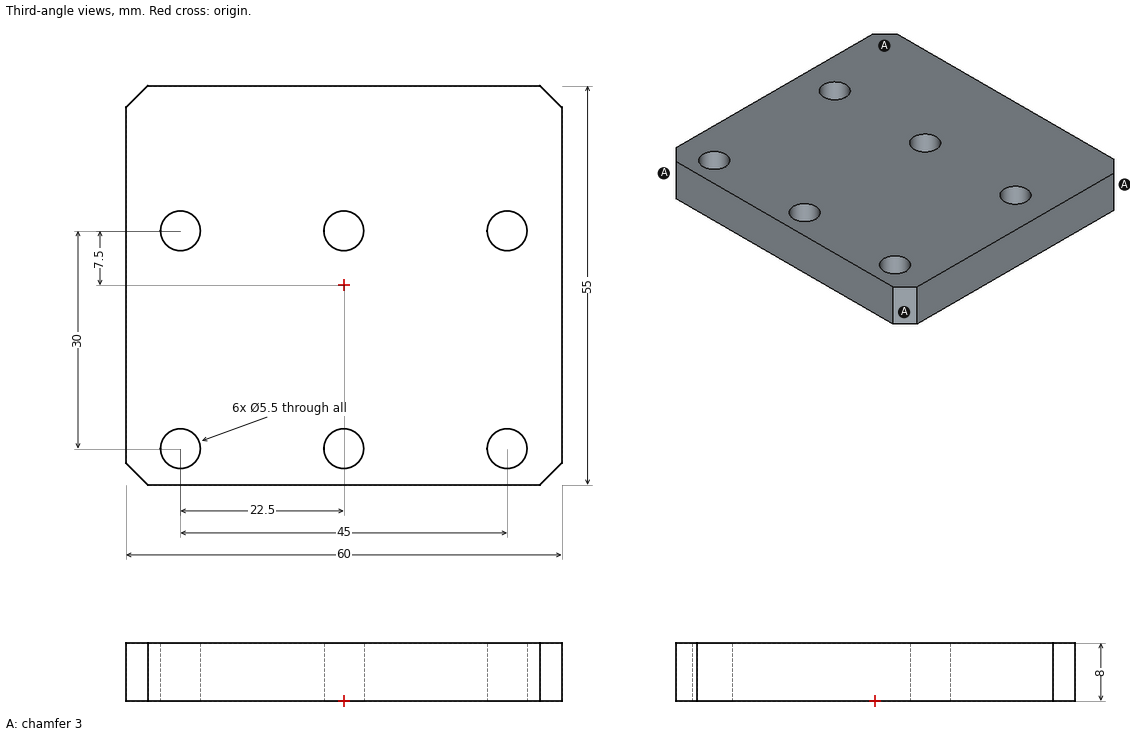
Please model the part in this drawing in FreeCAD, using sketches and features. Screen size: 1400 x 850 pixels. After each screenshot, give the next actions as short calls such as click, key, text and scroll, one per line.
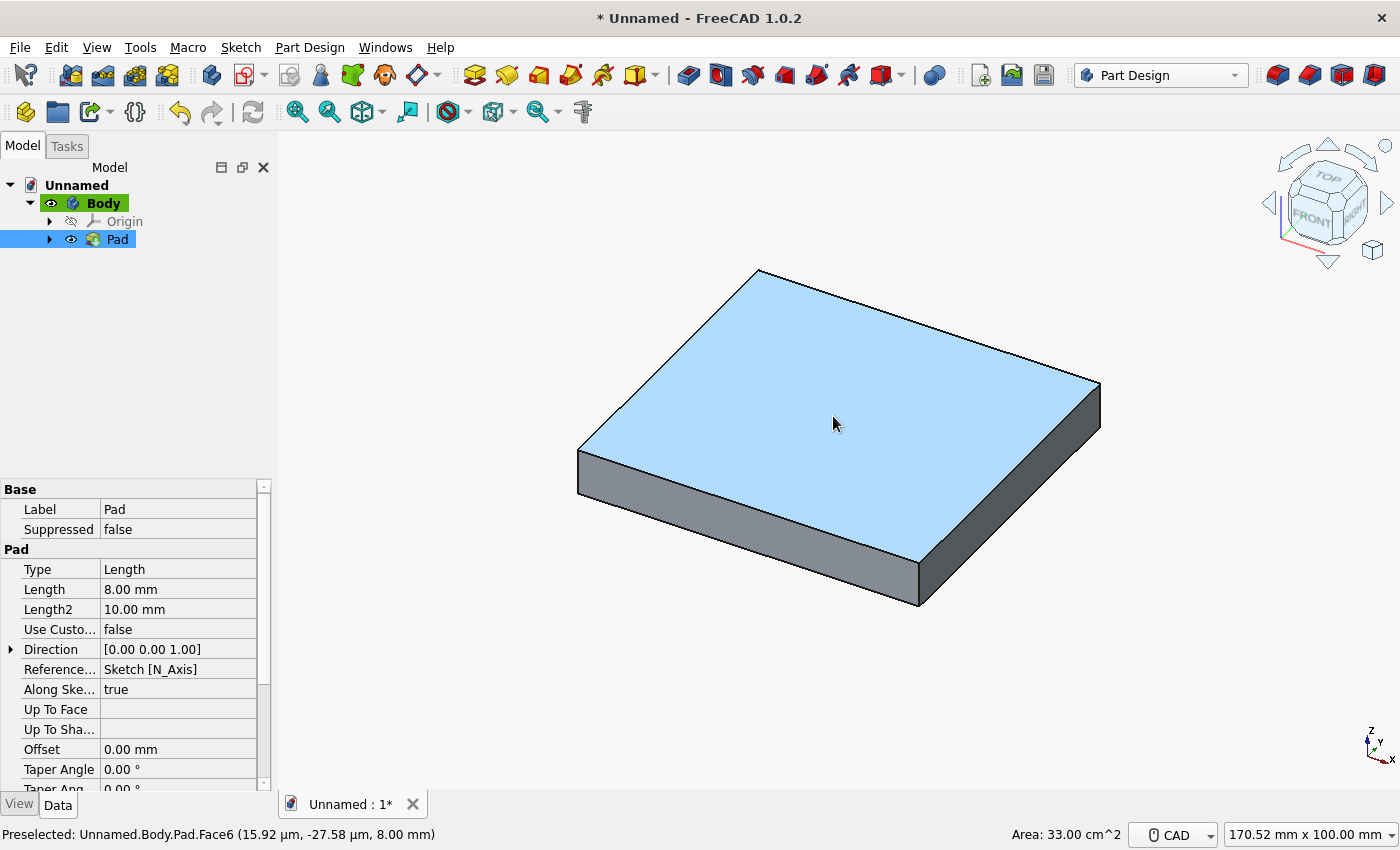
click(244, 76)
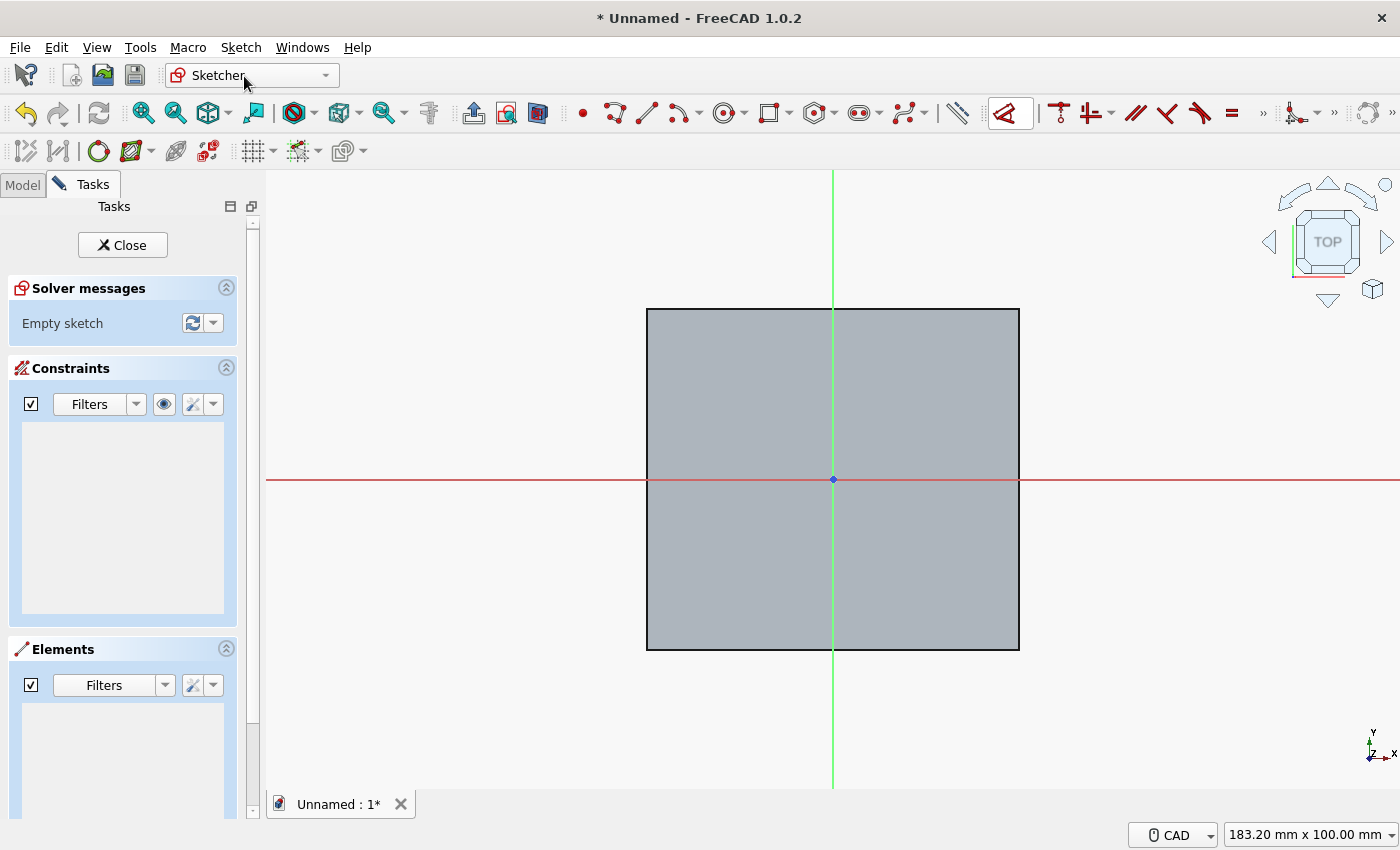
scroll(916, 582, up, 3)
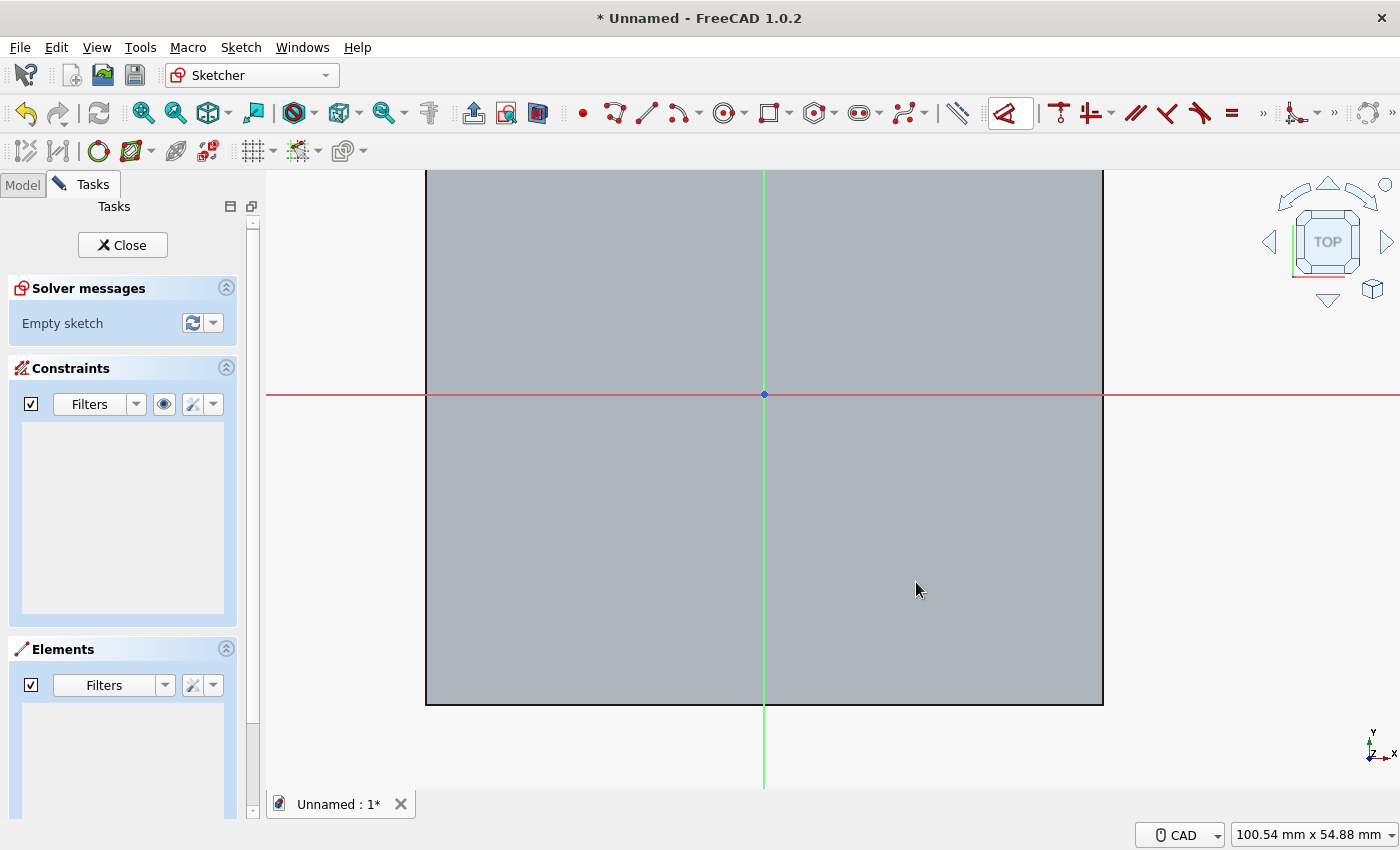
click(724, 114)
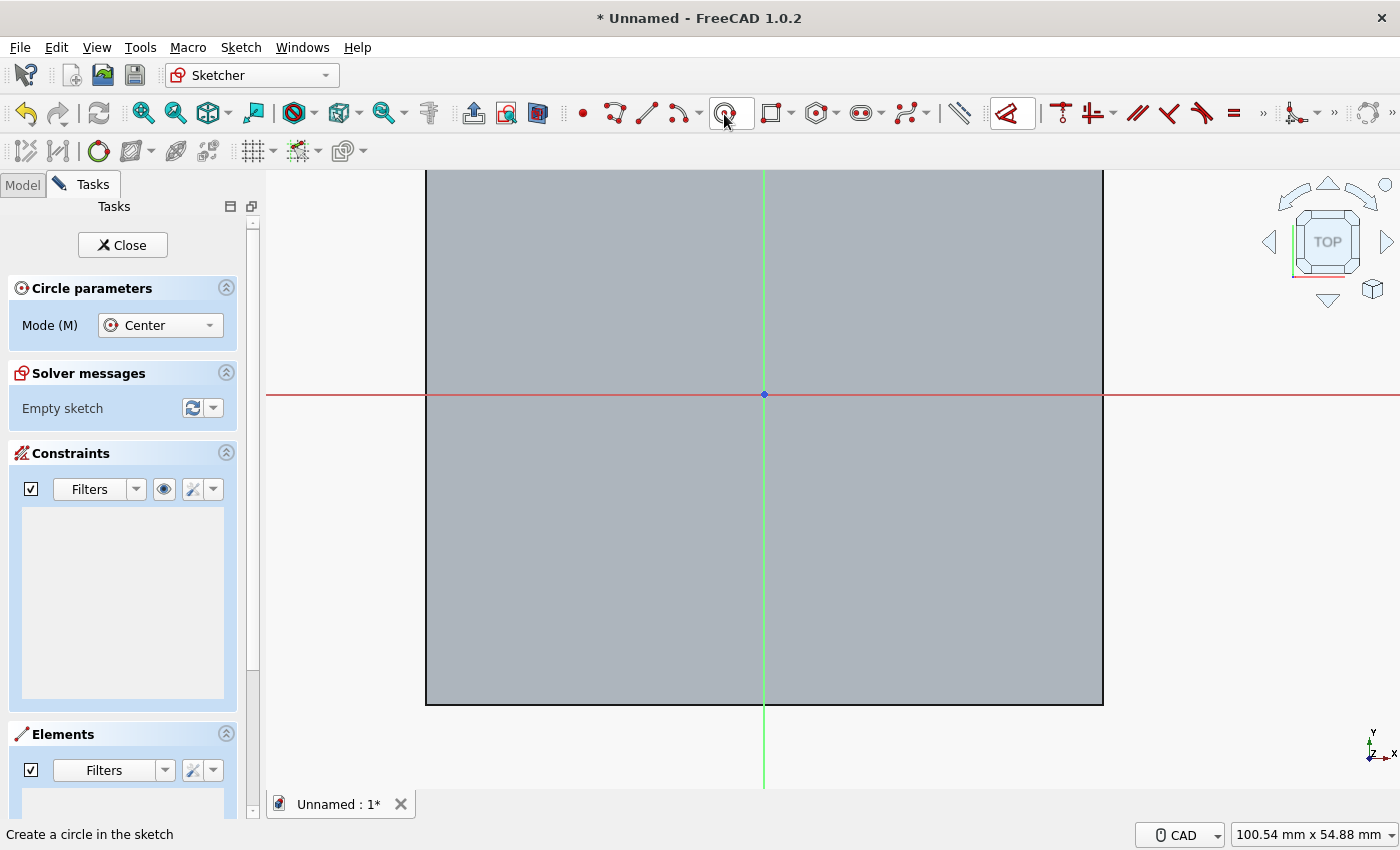
click(511, 648)
click(532, 627)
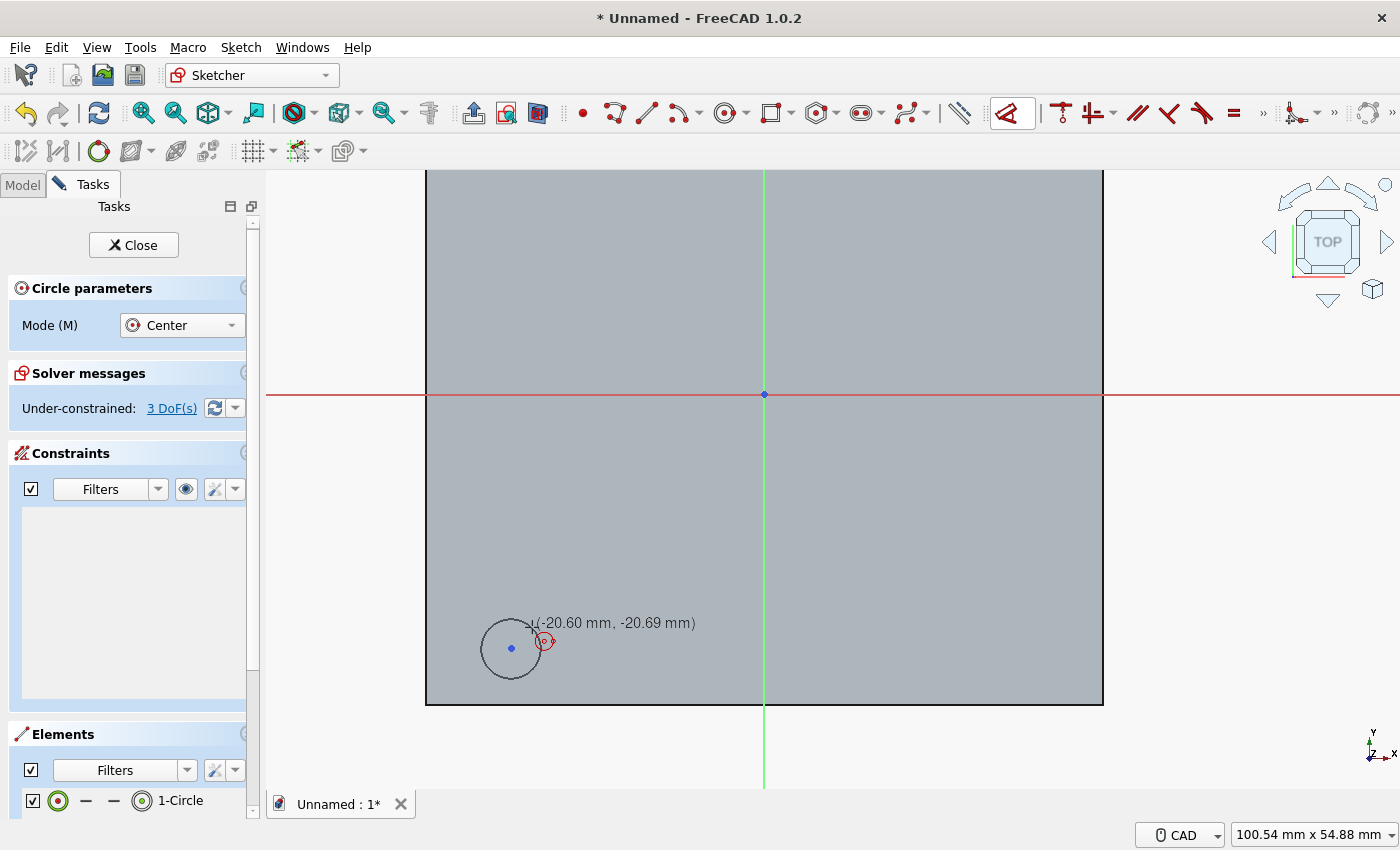
click(511, 310)
click(532, 288)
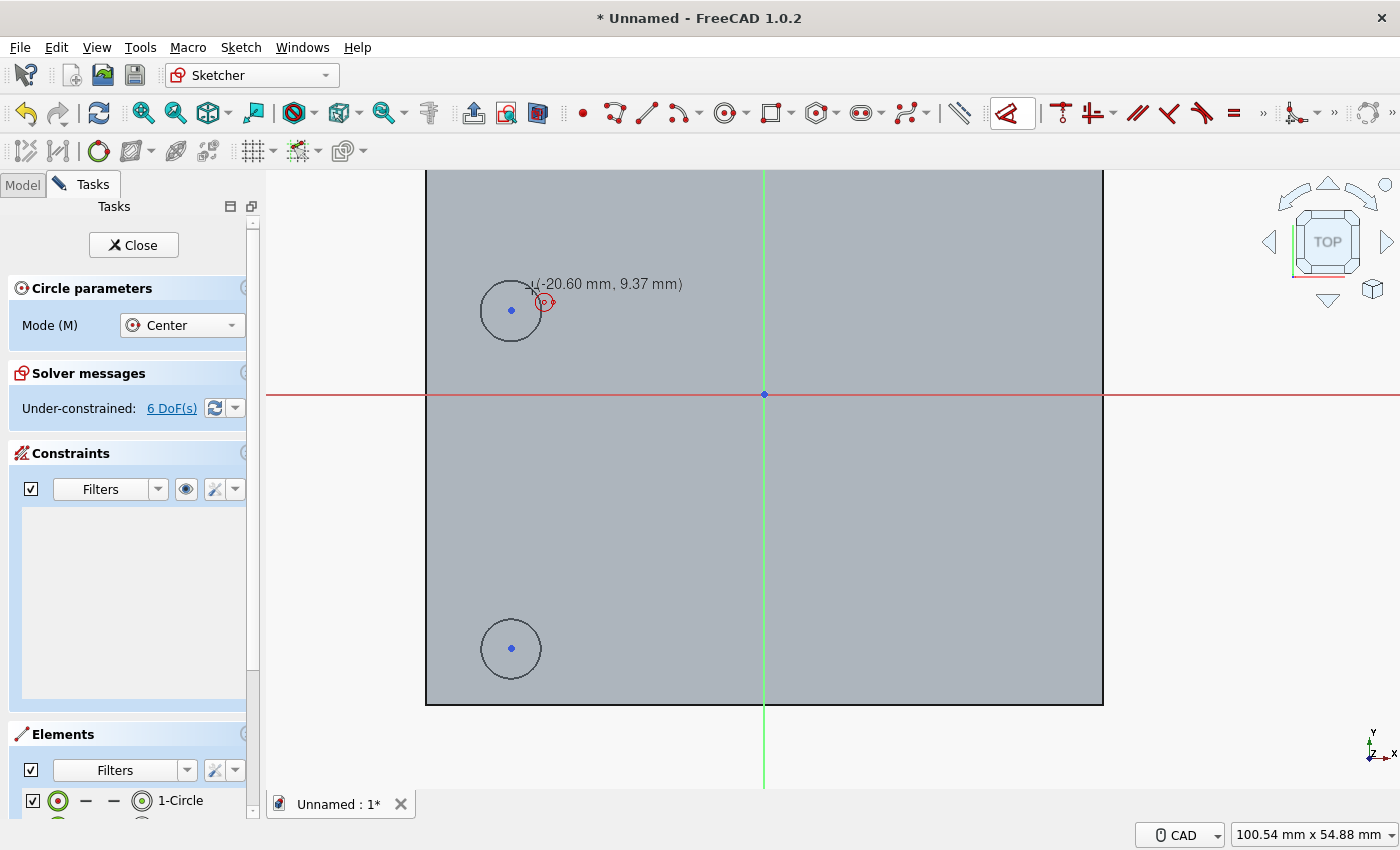
click(764, 310)
click(786, 288)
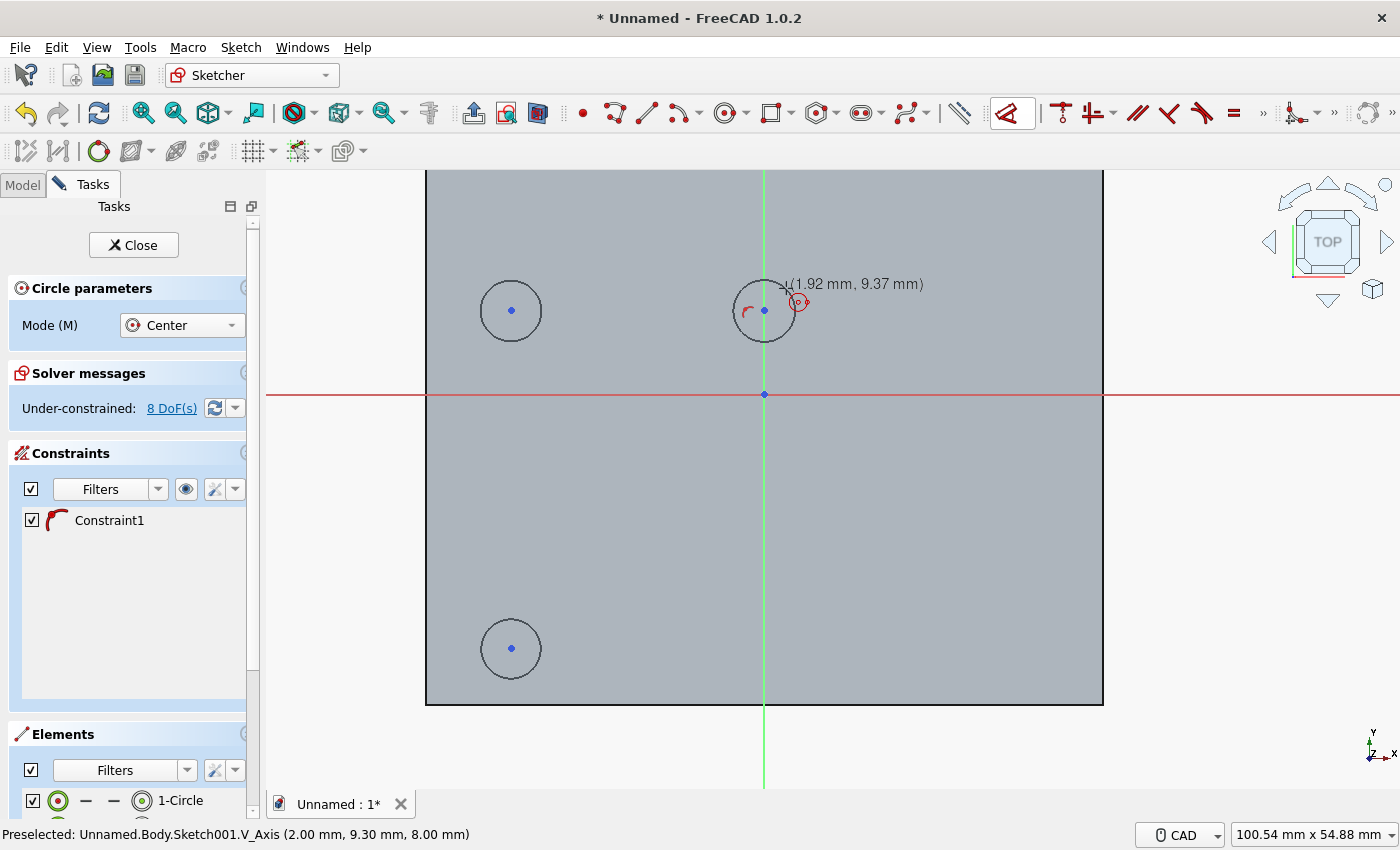
click(764, 648)
click(786, 627)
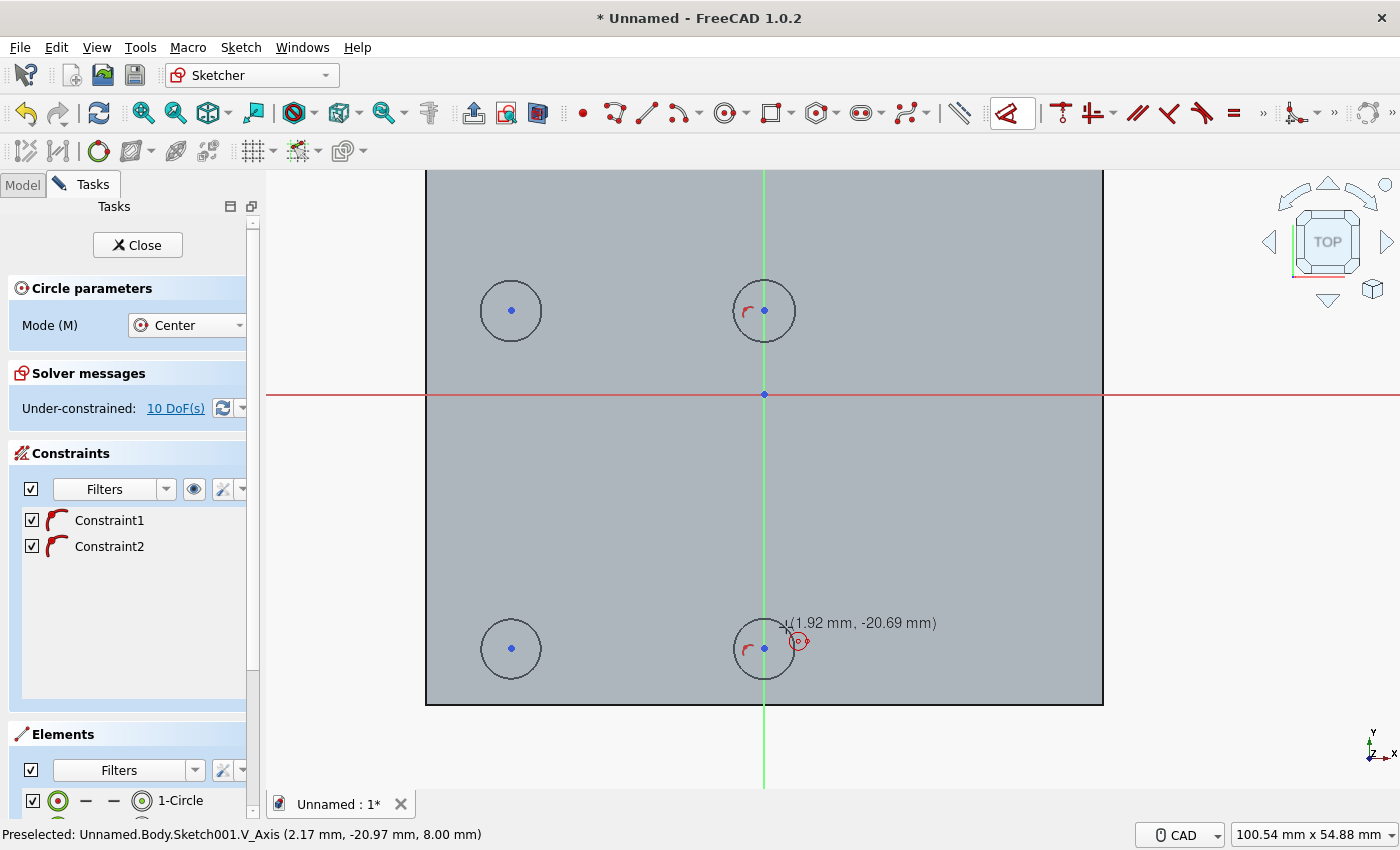
click(1018, 648)
click(1040, 627)